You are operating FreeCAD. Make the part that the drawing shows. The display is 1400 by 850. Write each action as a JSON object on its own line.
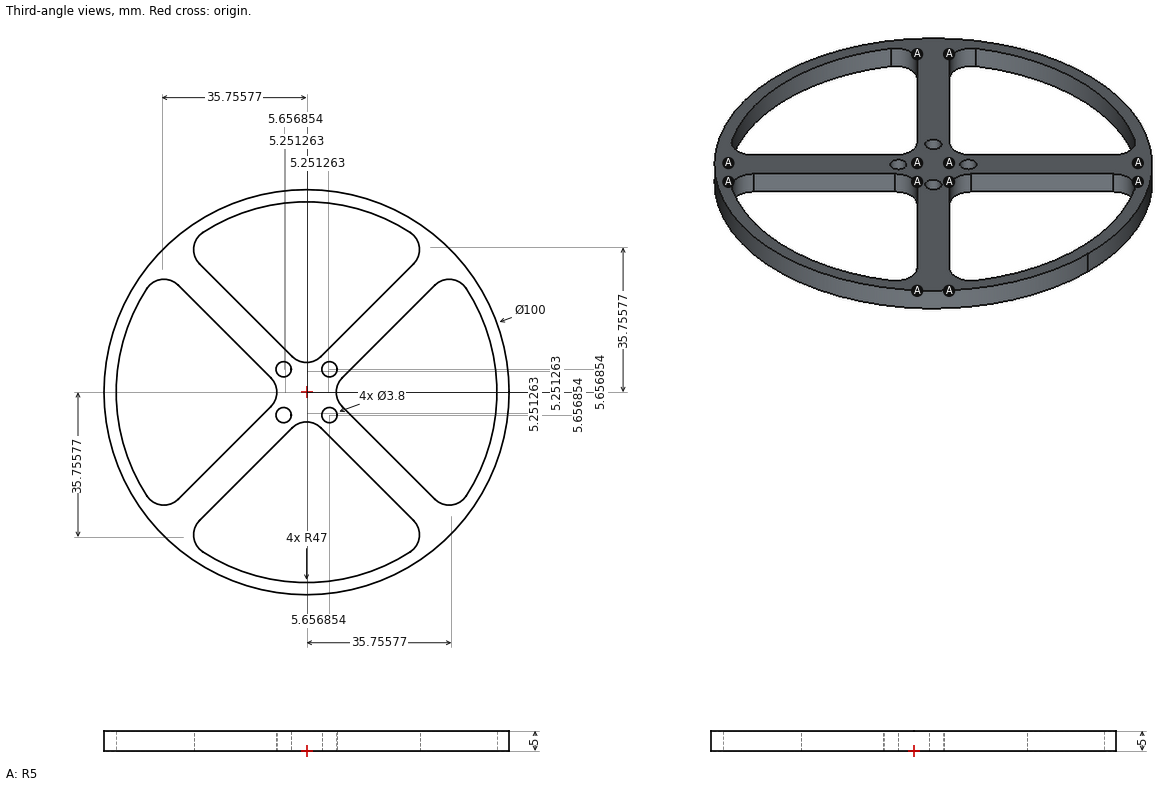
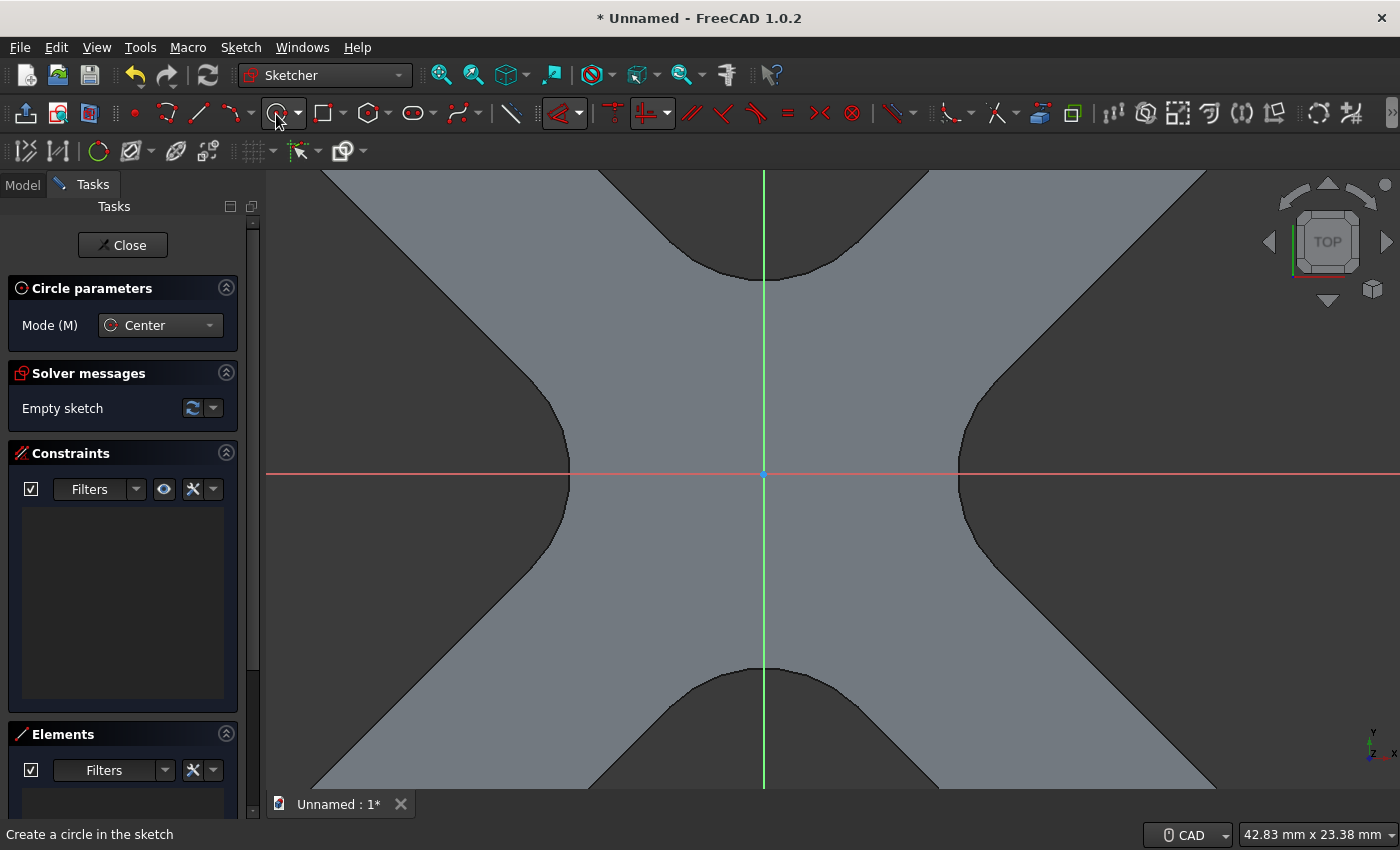
{"action": "left_click", "coordinate": [914, 624]}
{"action": "mouse_move", "coordinate": [949, 589]}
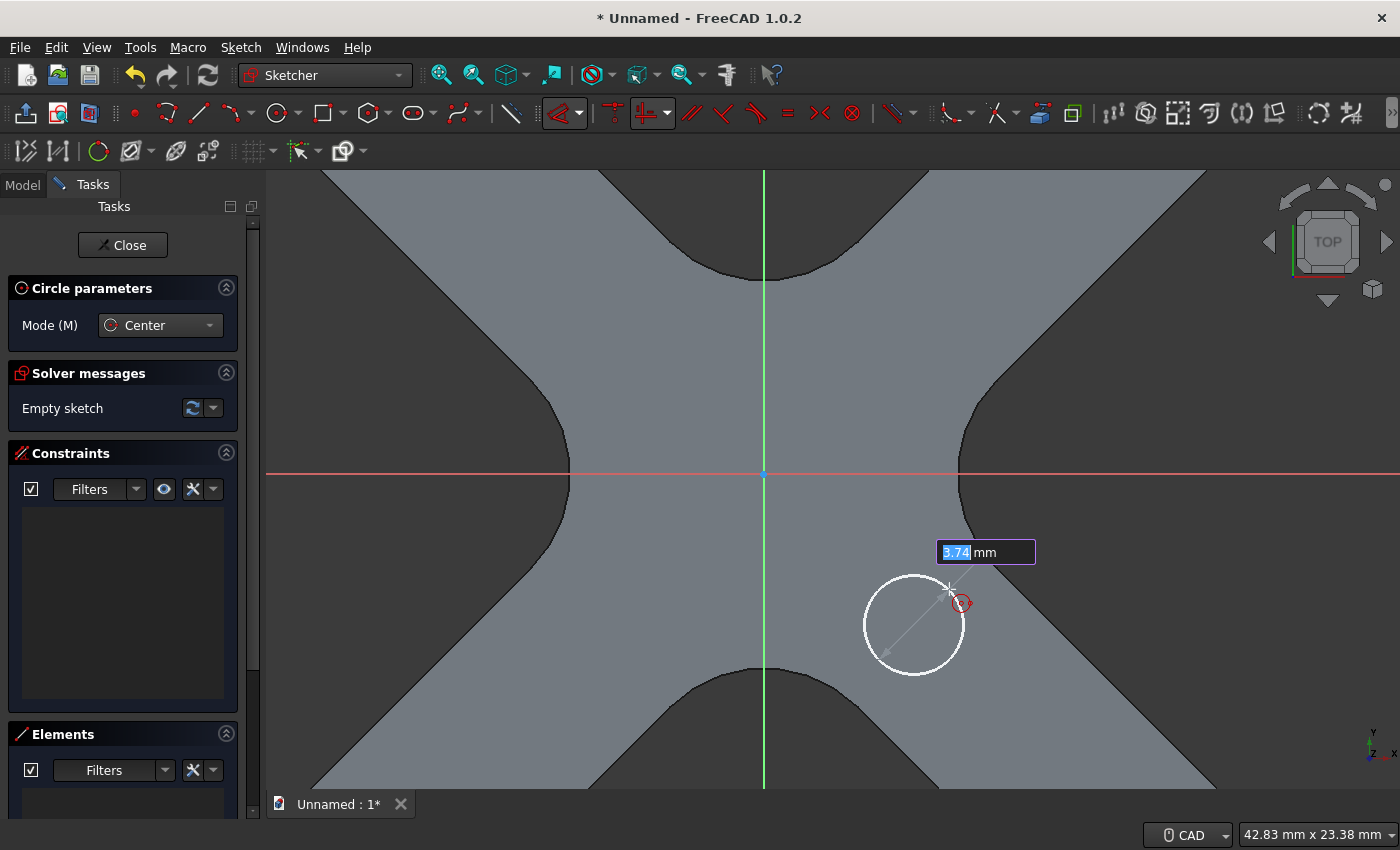
{"action": "type", "text": "3.8"}
{"action": "key", "text": "Return"}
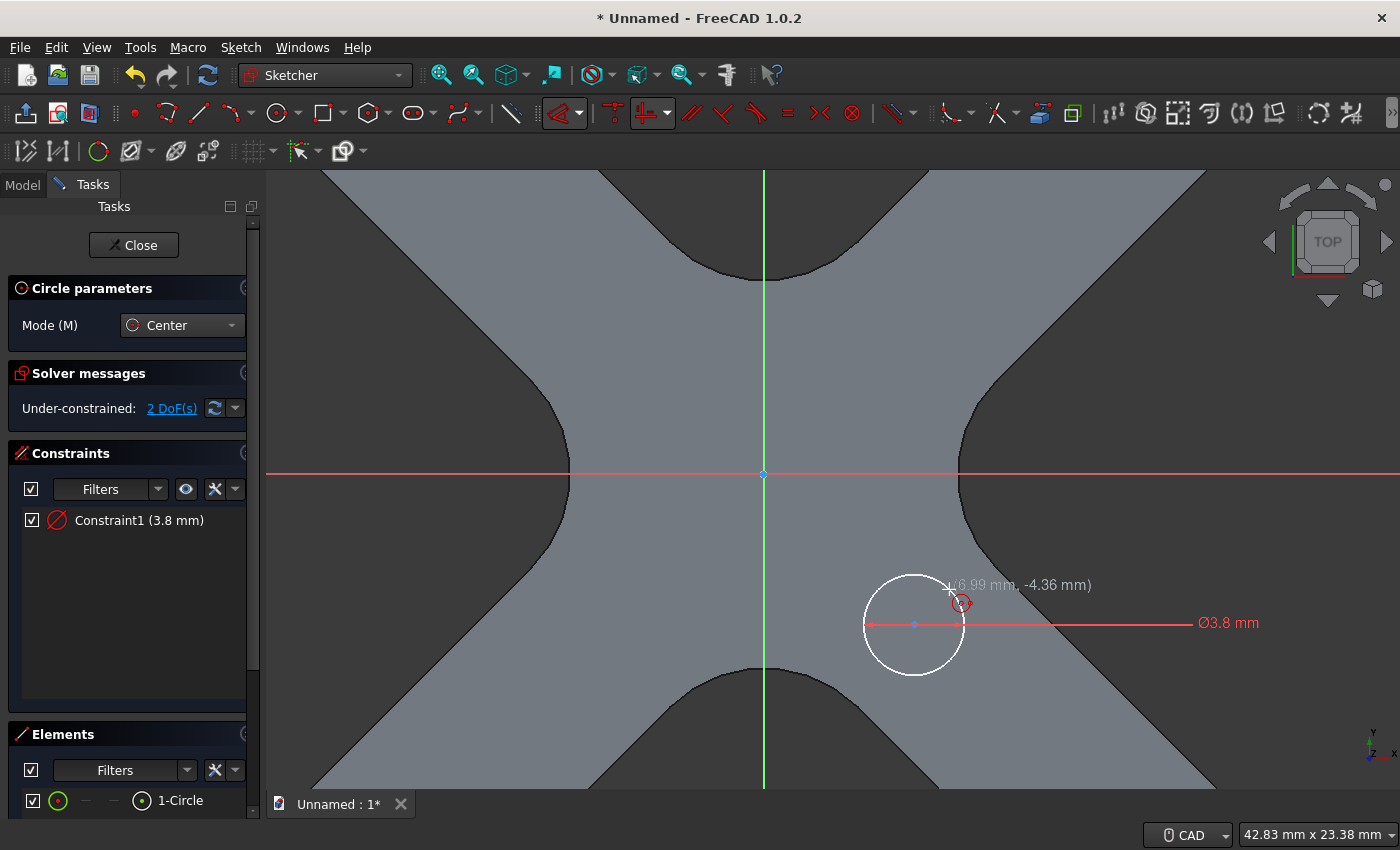
{"action": "left_click", "coordinate": [914, 325]}
{"action": "mouse_move", "coordinate": [949, 289]}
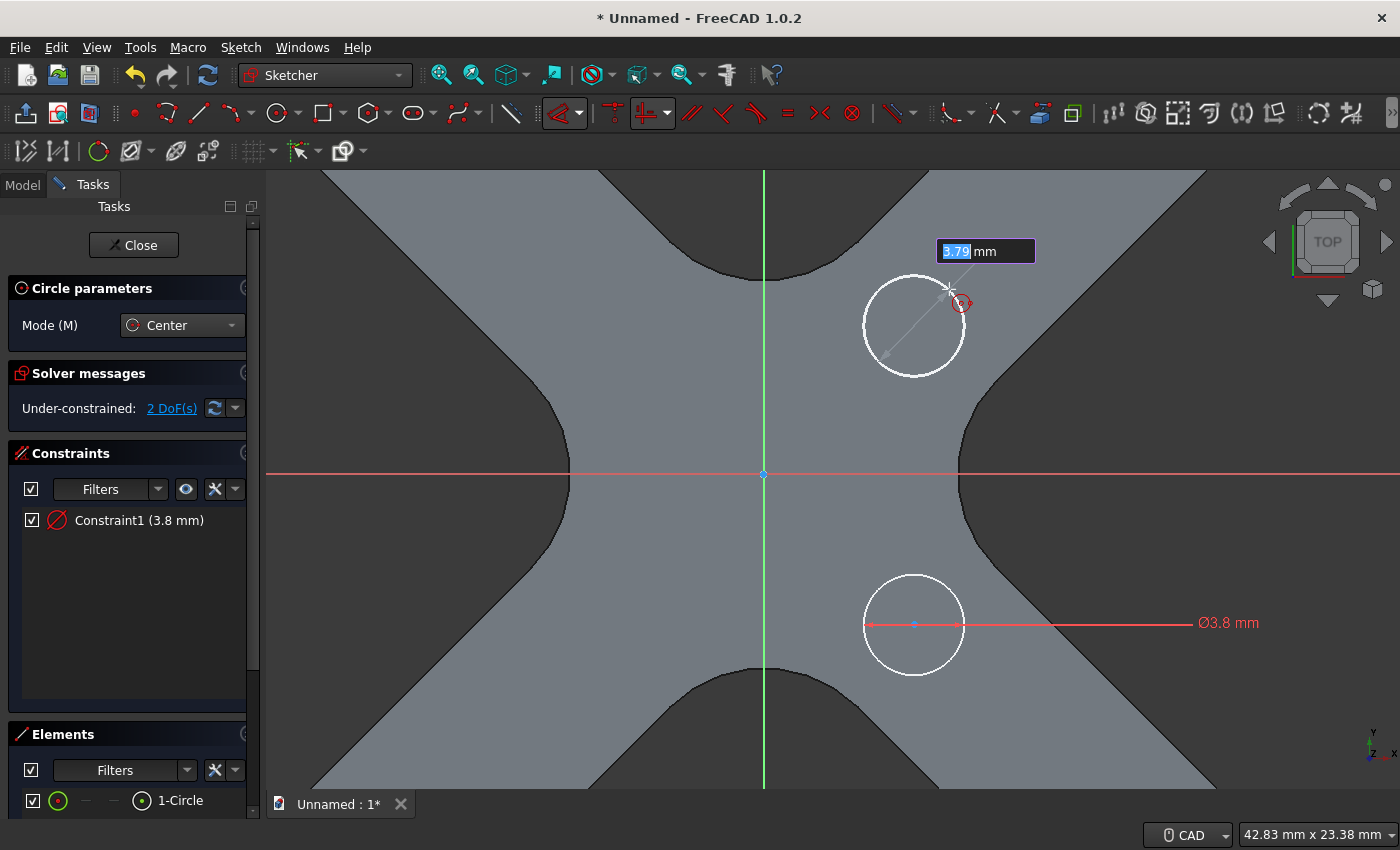
{"action": "type", "text": "3.8"}
{"action": "key", "text": "Return"}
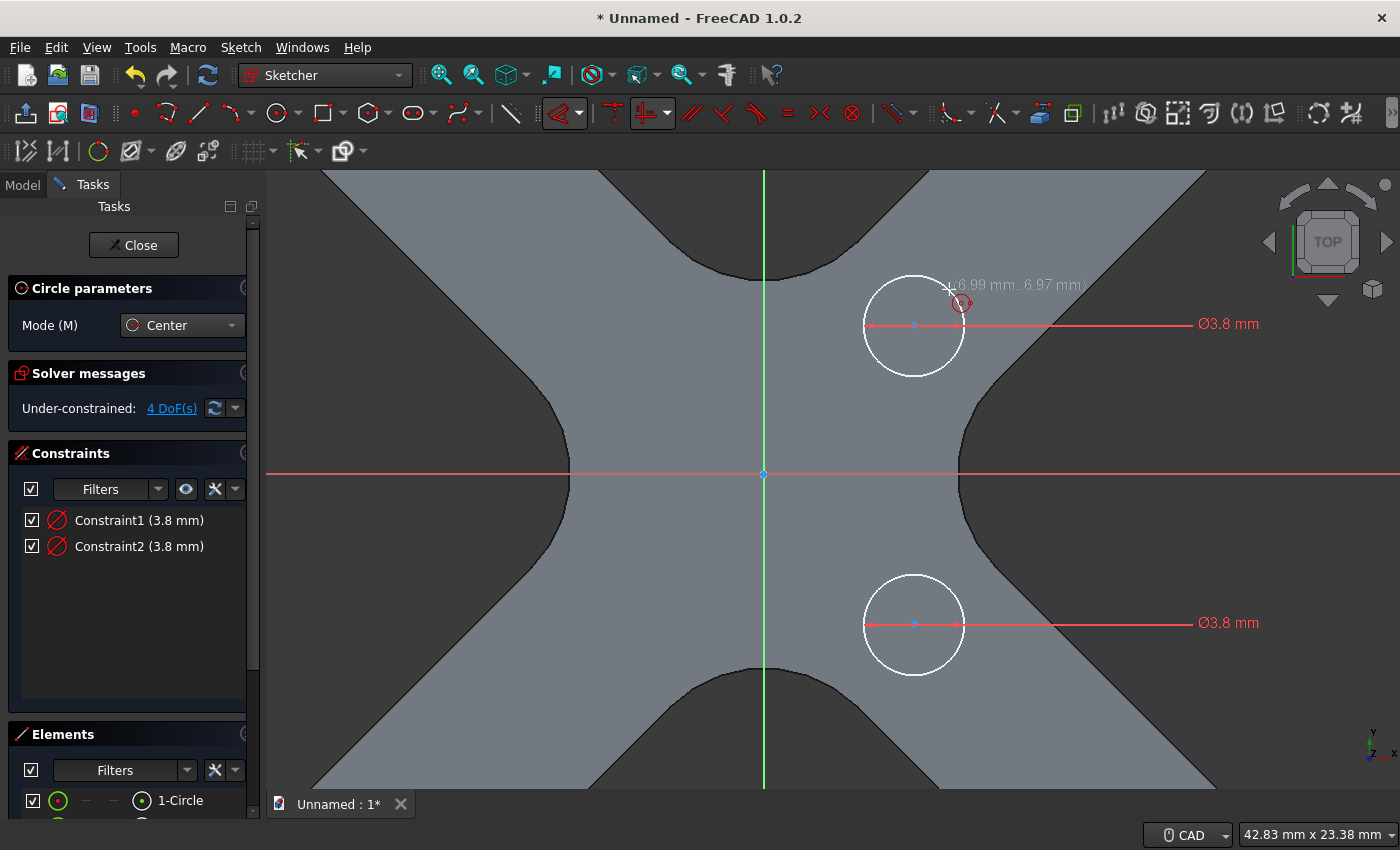
{"action": "left_click", "coordinate": [614, 325]}
{"action": "mouse_move", "coordinate": [650, 289]}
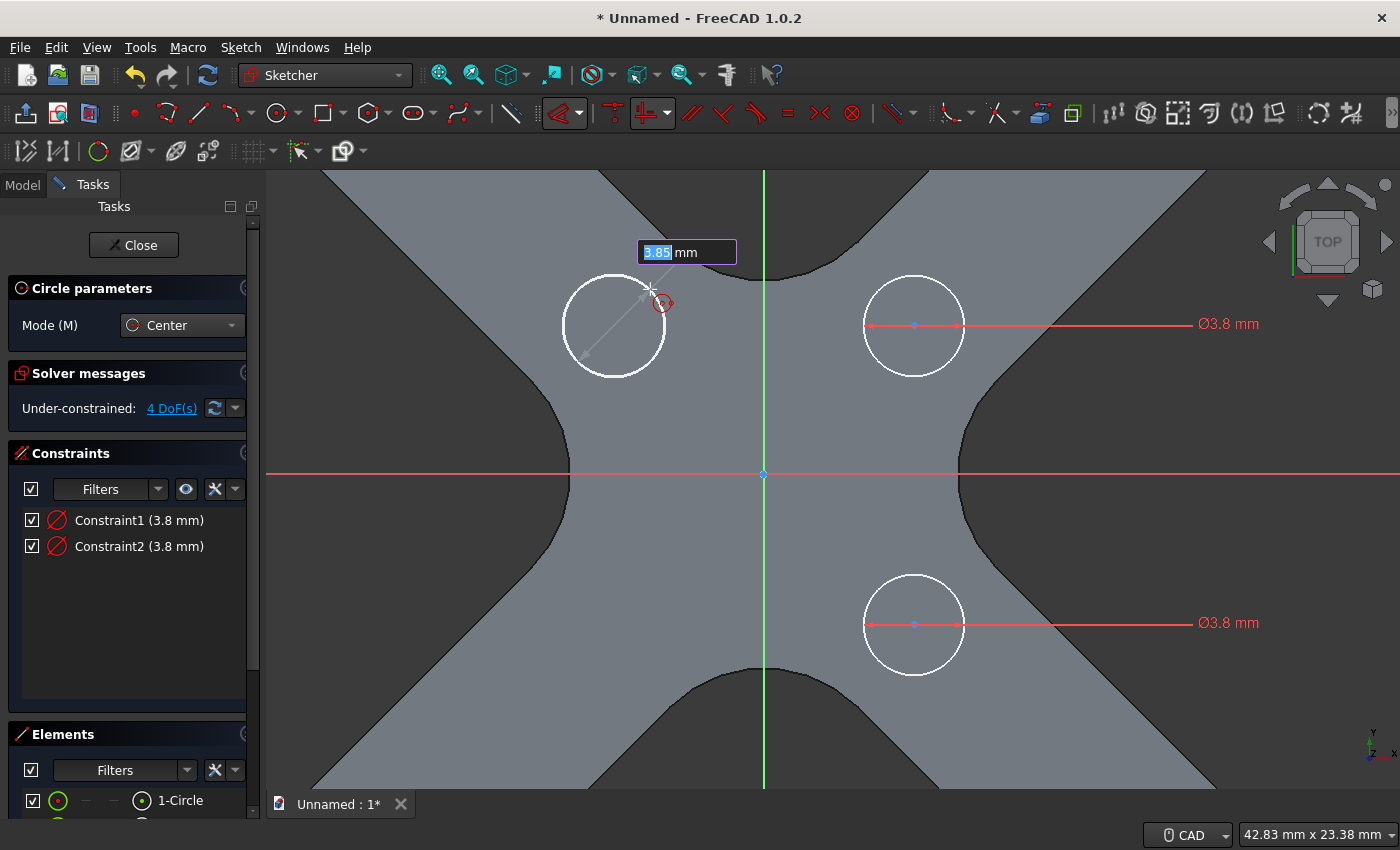
{"action": "type", "text": "3.8"}
{"action": "key", "text": "Return"}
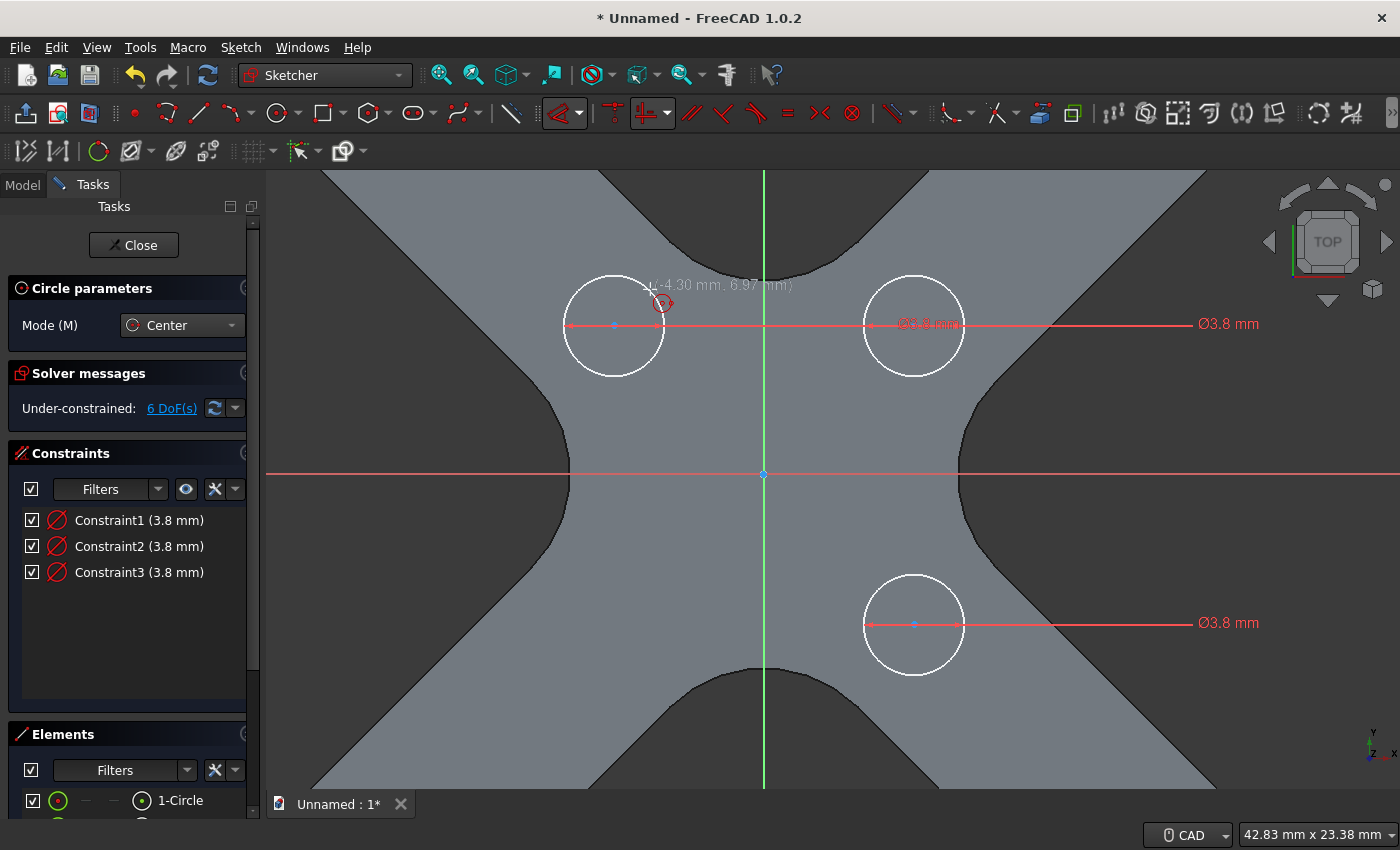
{"action": "left_click", "coordinate": [614, 624]}
{"action": "mouse_move", "coordinate": [650, 589]}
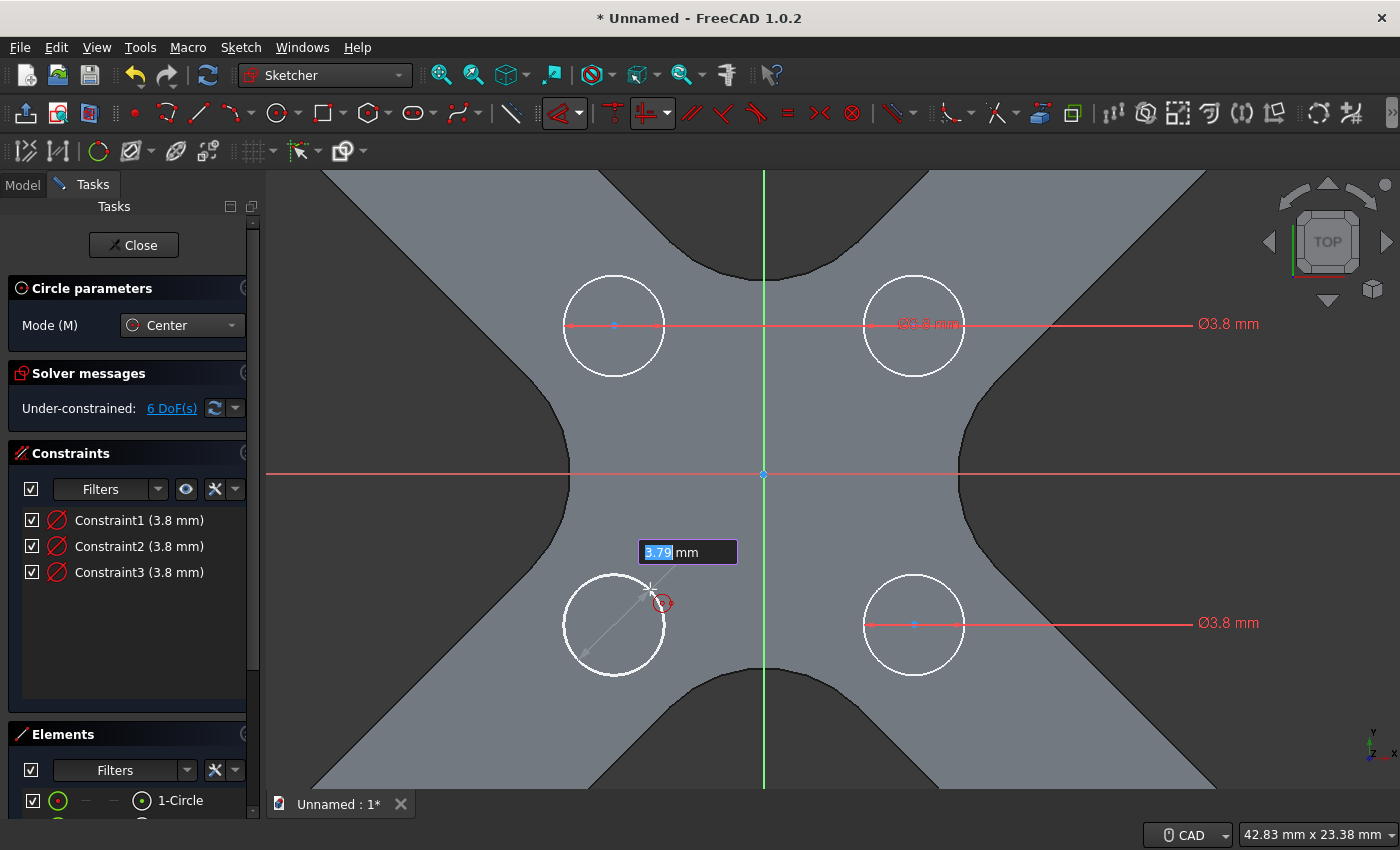
{"action": "type", "text": "3.8"}
{"action": "key", "text": "Return"}
{"action": "key", "text": "Escape"}